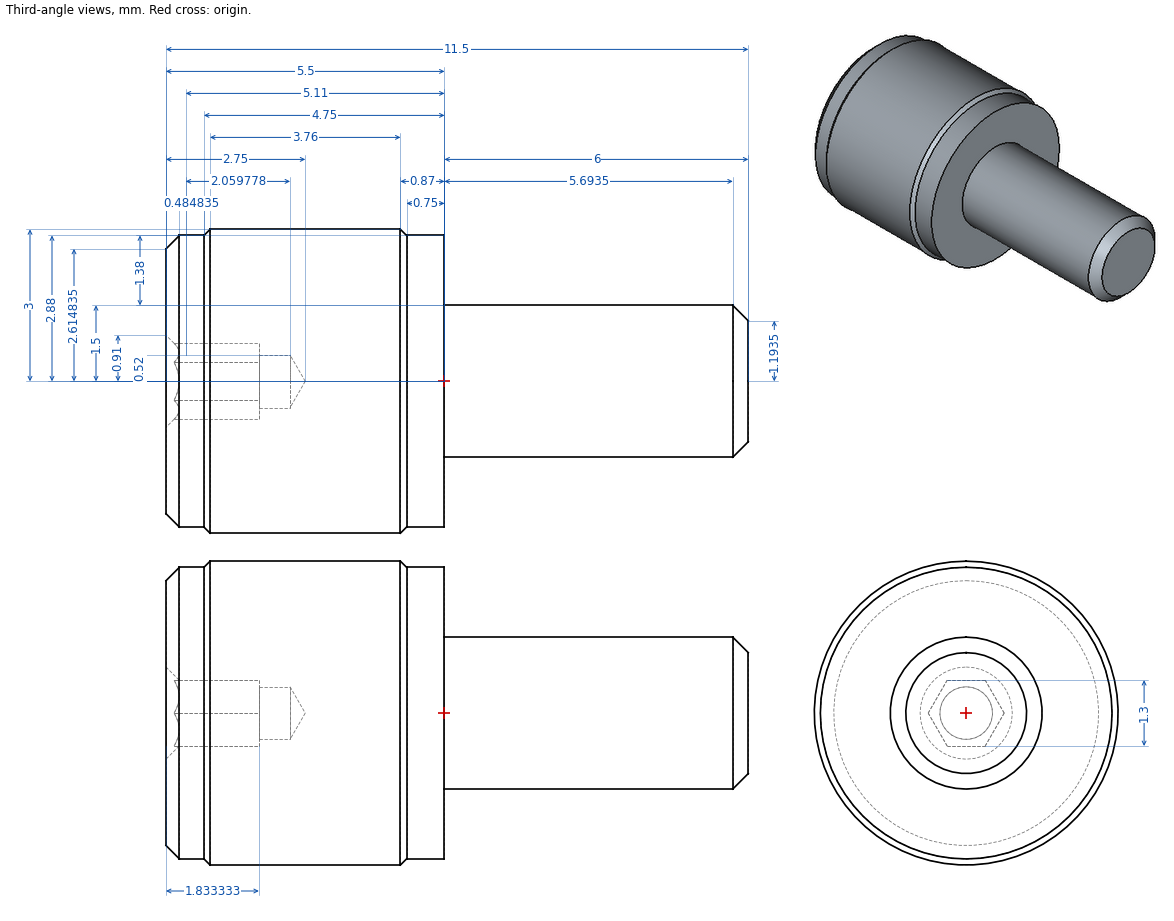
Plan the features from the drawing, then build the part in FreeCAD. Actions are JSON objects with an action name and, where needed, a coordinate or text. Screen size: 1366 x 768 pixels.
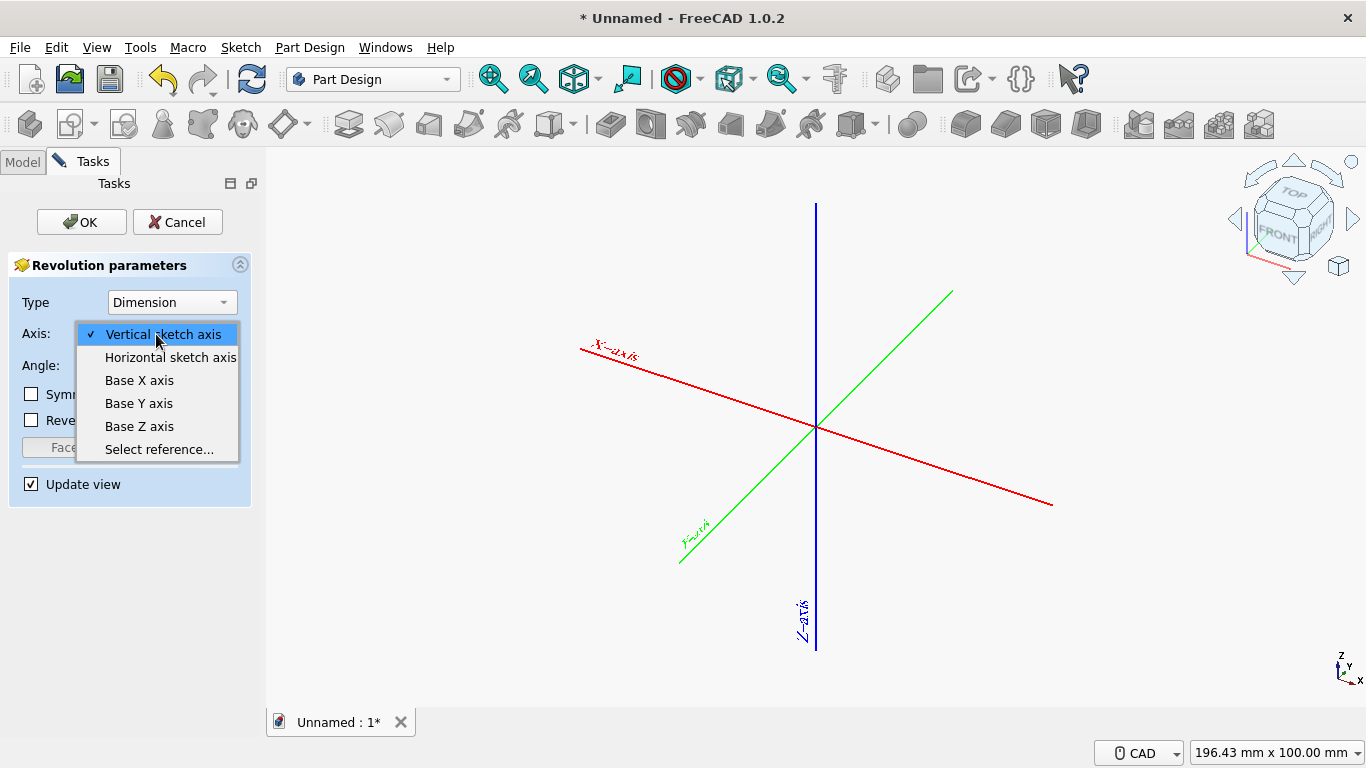
{"action": "left_click", "coordinate": [156, 358]}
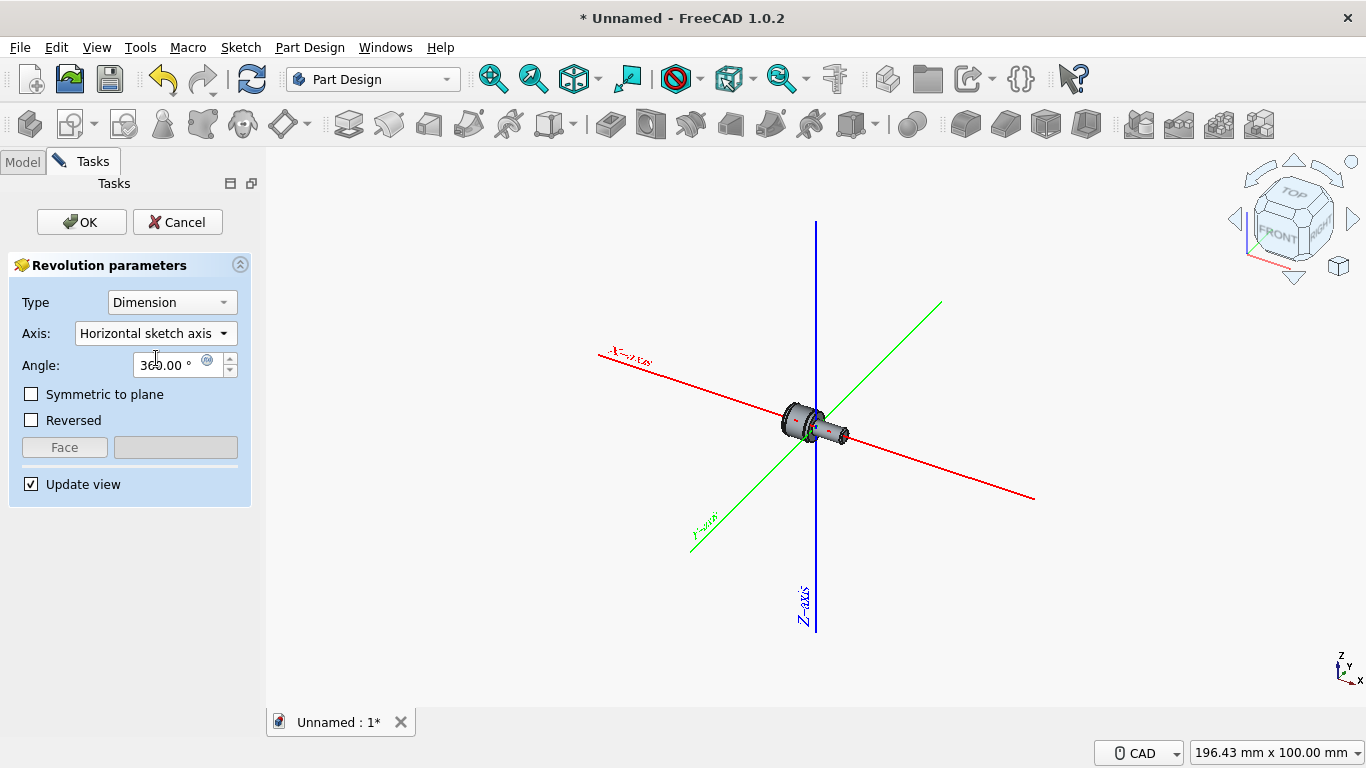
{"action": "left_click", "coordinate": [82, 222]}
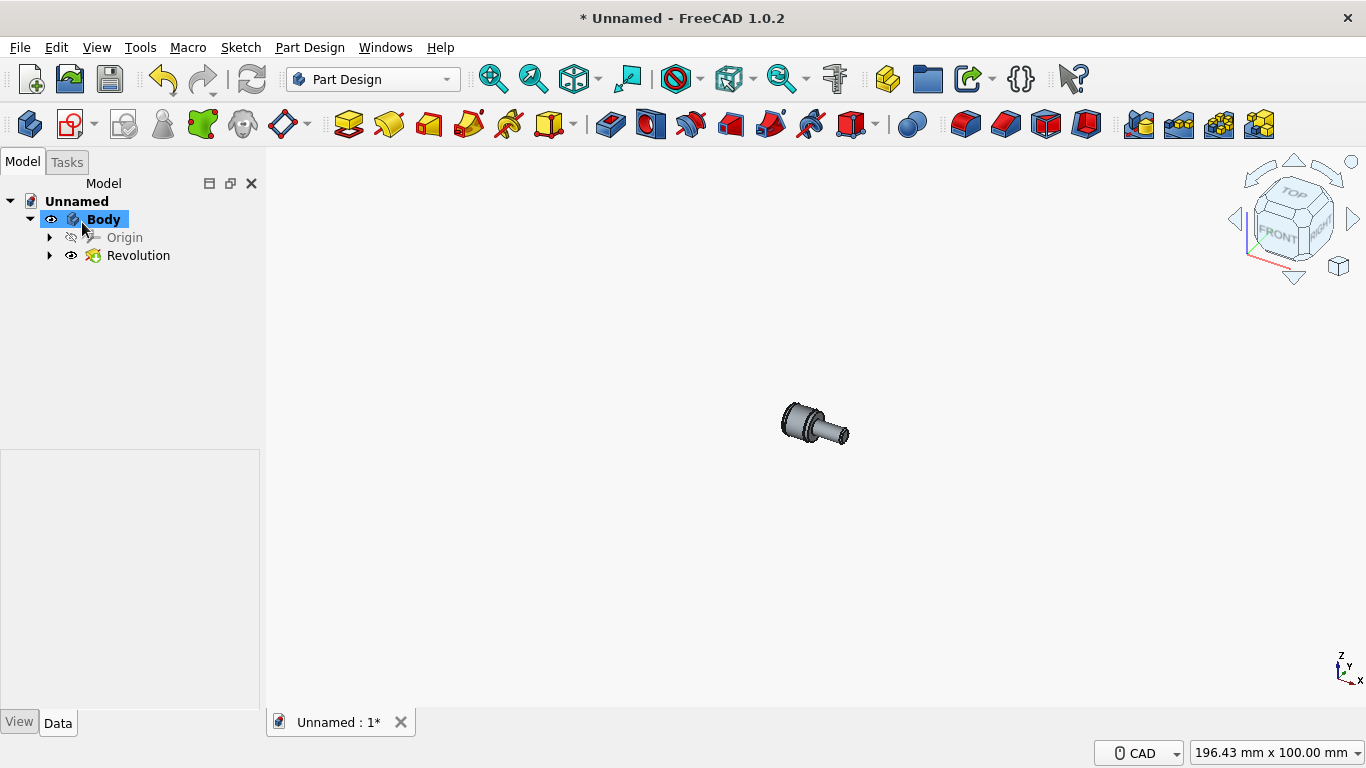
{"action": "key", "text": "v f"}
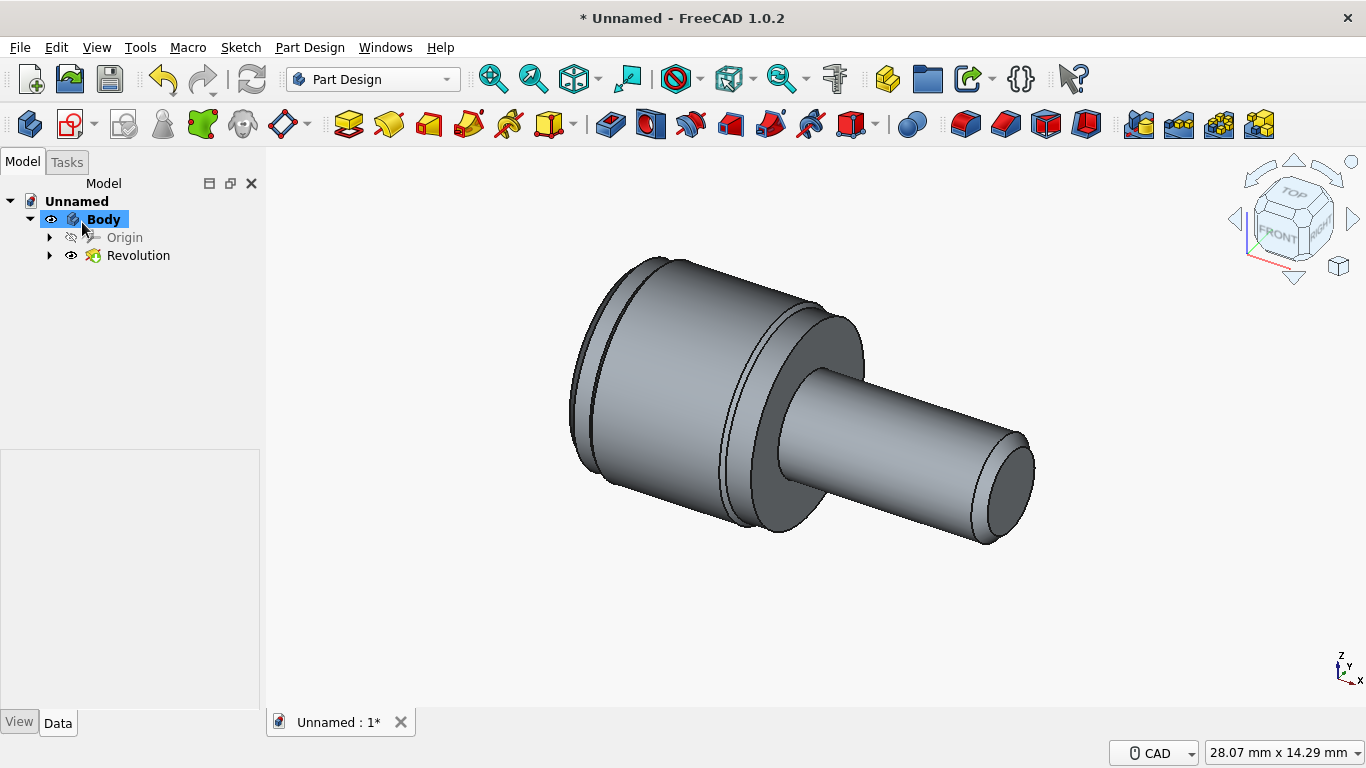
{"action": "left_click", "coordinate": [70, 124]}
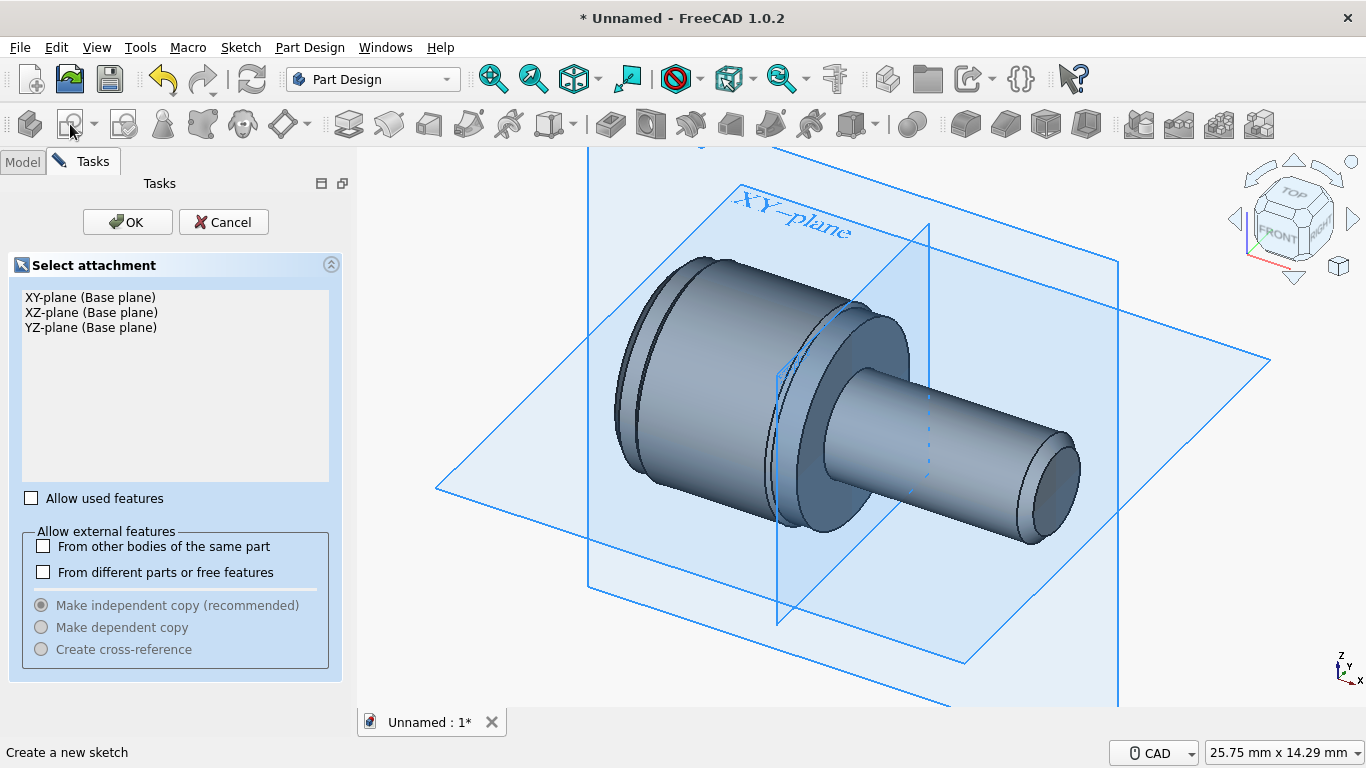
{"action": "left_click", "coordinate": [82, 298]}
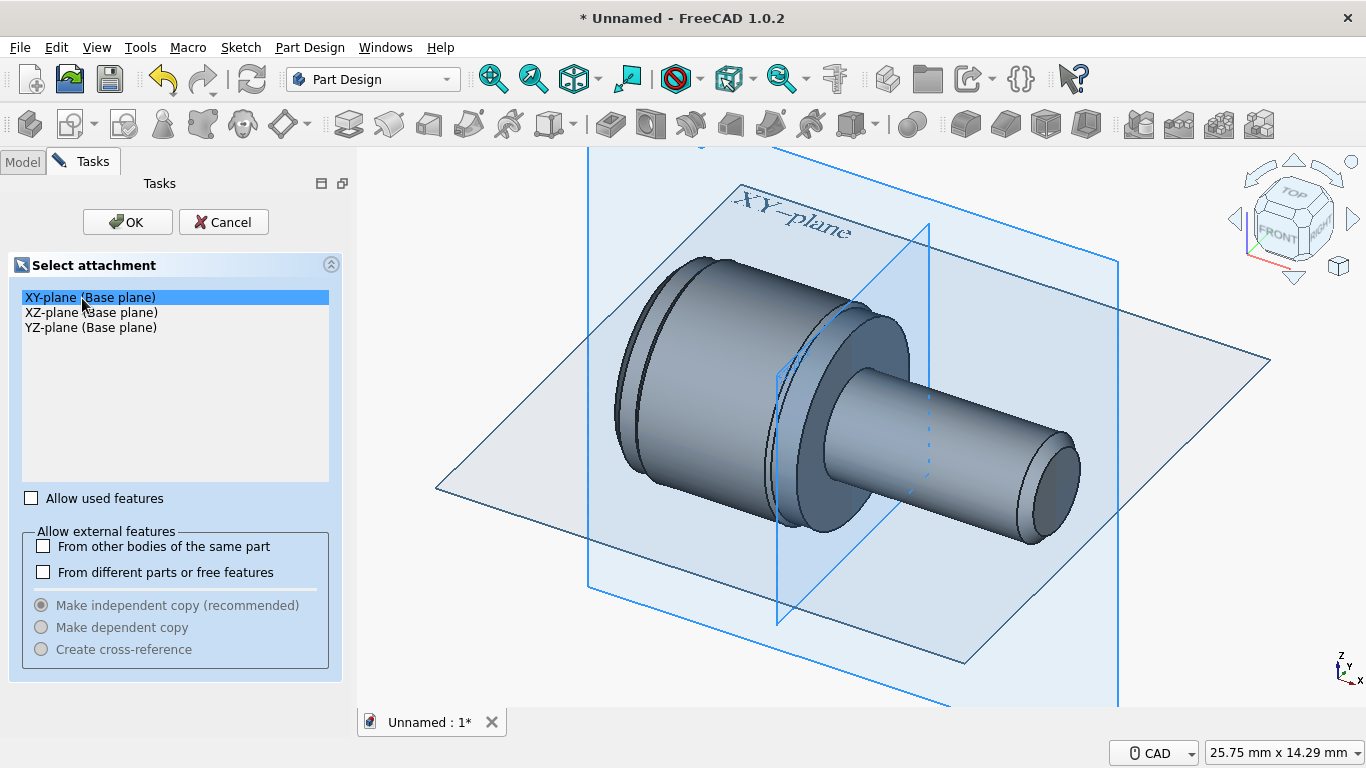
{"action": "left_click", "coordinate": [128, 222]}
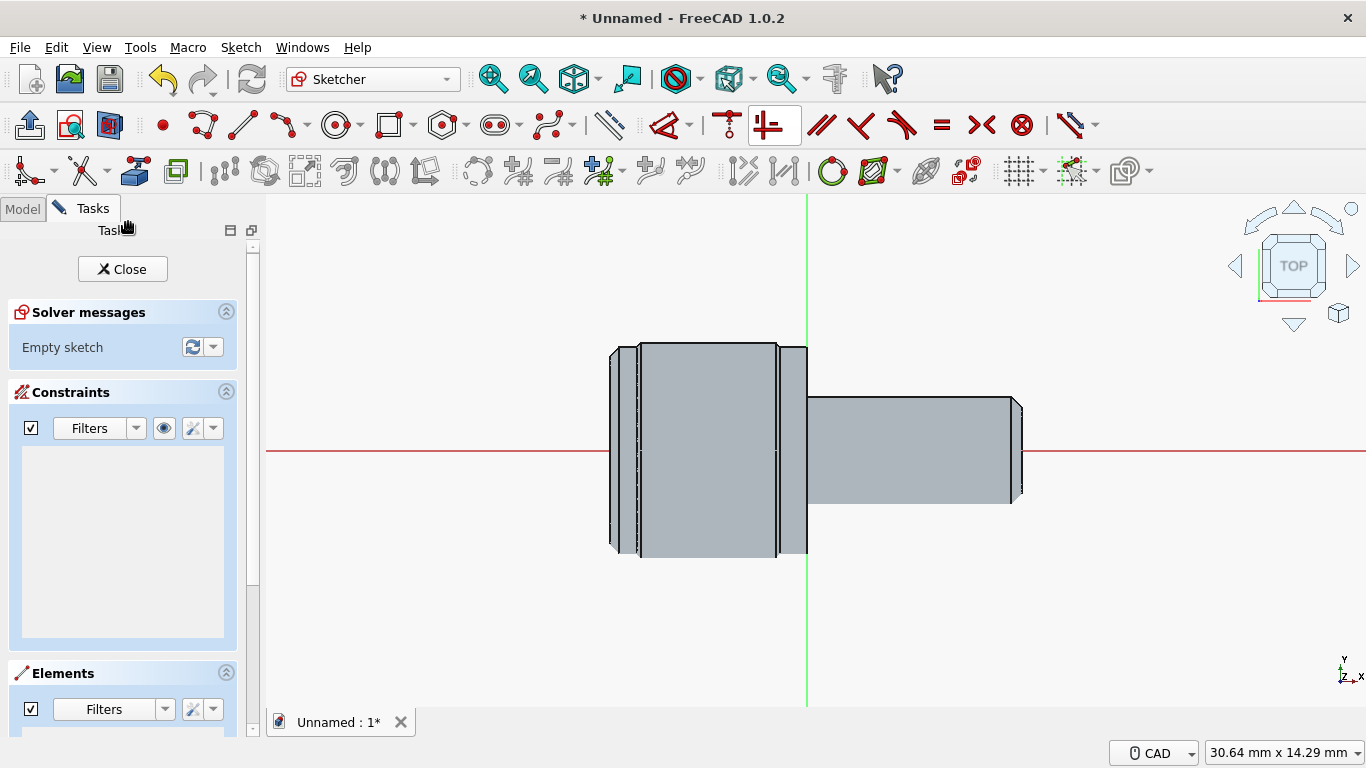
{"action": "left_click", "coordinate": [110, 126]}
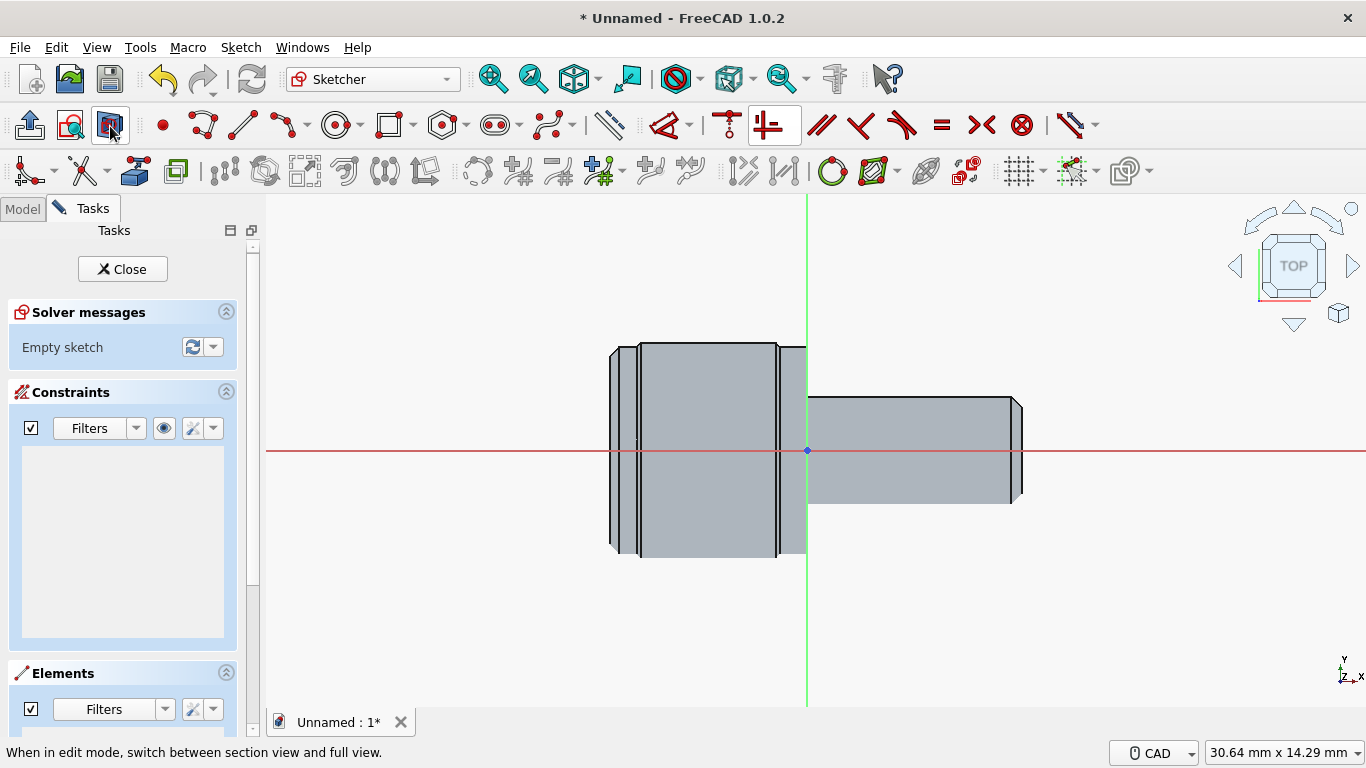
{"action": "scroll", "coordinate": [691, 427], "scroll_direction": "up", "scroll_amount": 6}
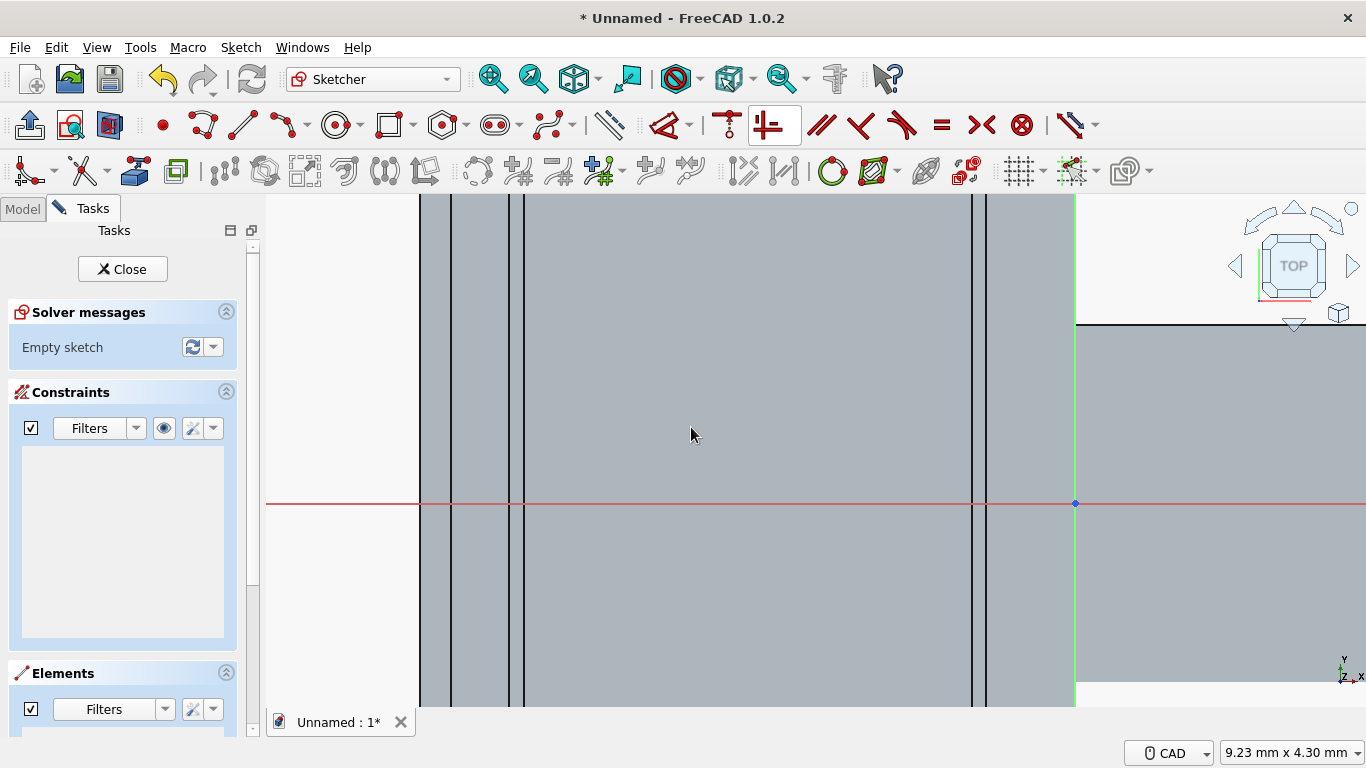
{"action": "left_click", "coordinate": [204, 126]}